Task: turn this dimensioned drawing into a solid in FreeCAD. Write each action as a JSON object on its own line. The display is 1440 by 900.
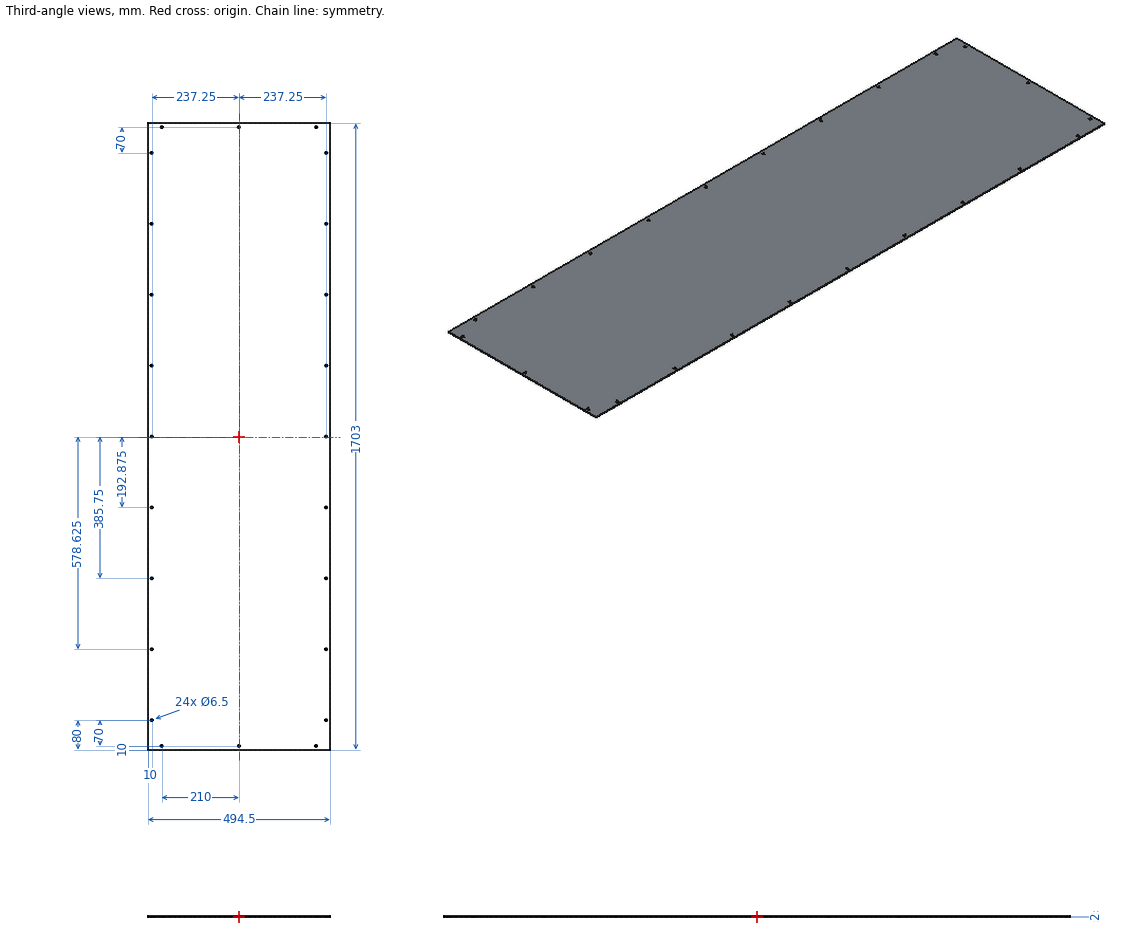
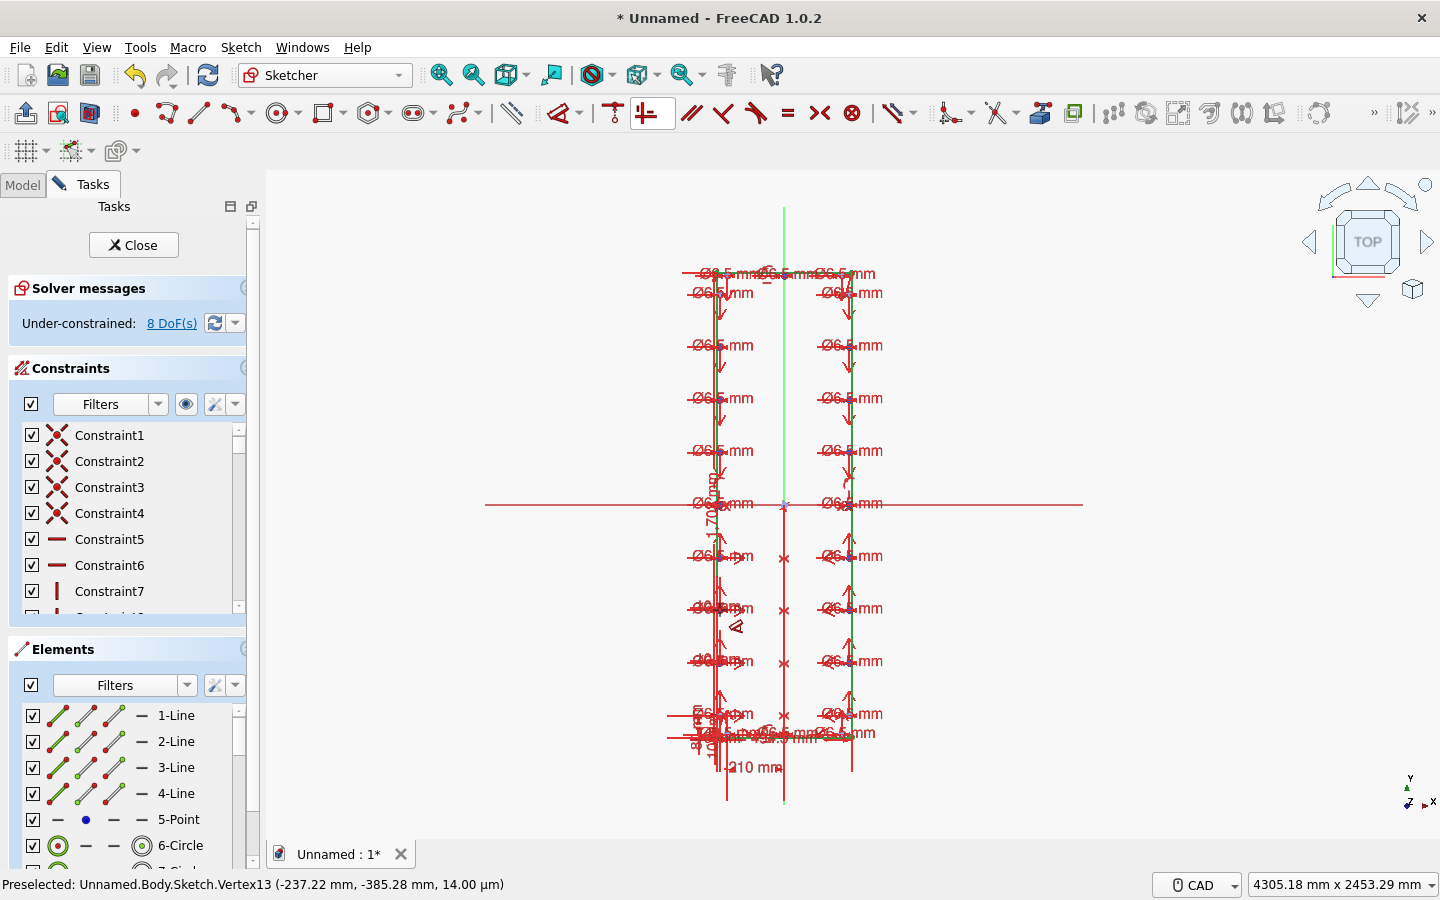
{"action": "scroll", "coordinate": [717, 738], "scroll_direction": "up", "scroll_amount": 14}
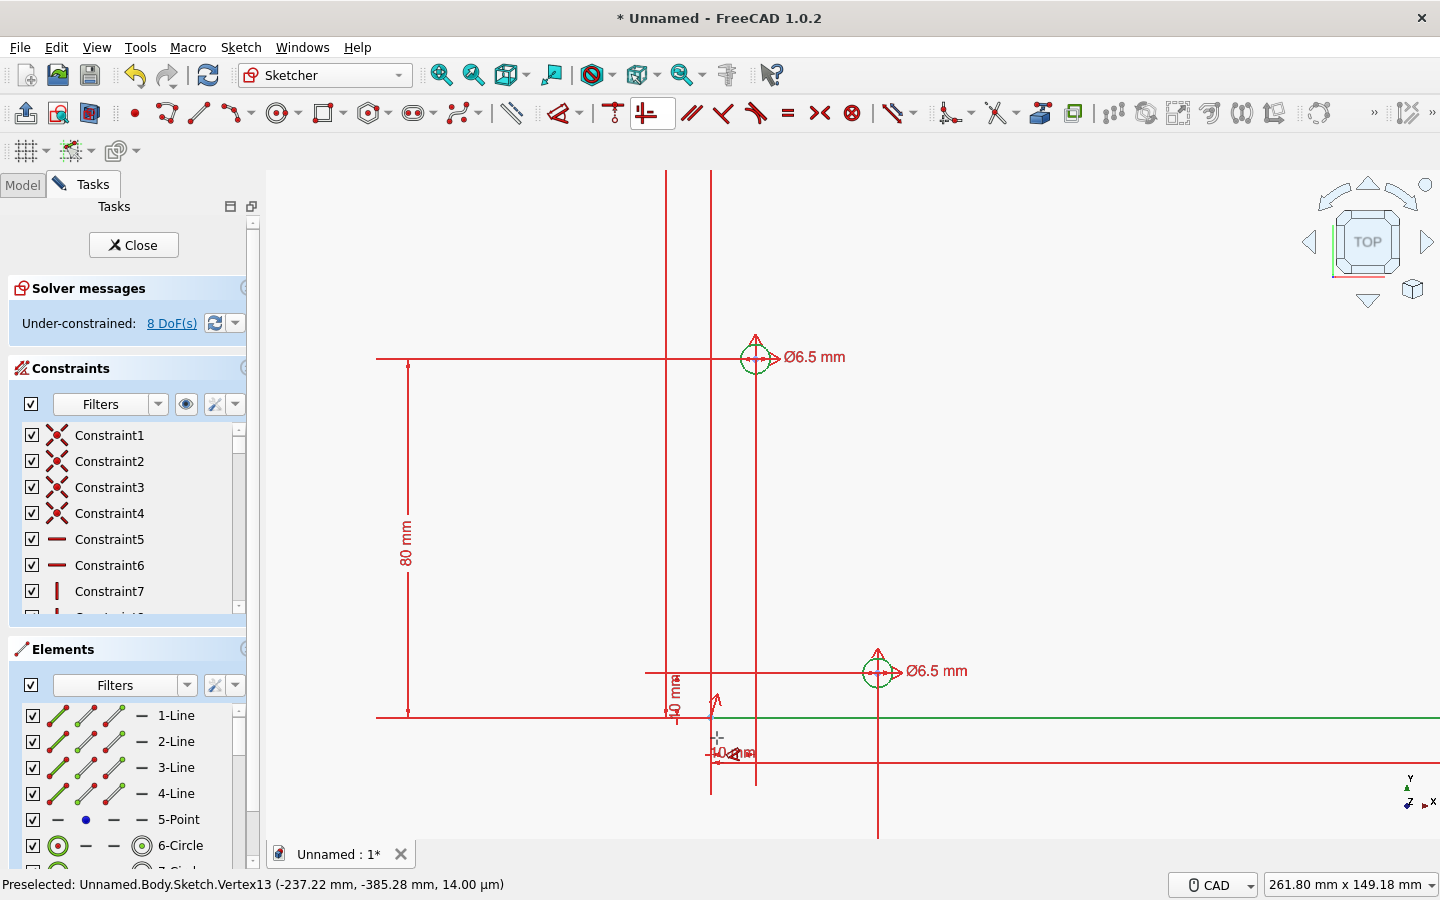
{"action": "left_click", "coordinate": [711, 718]}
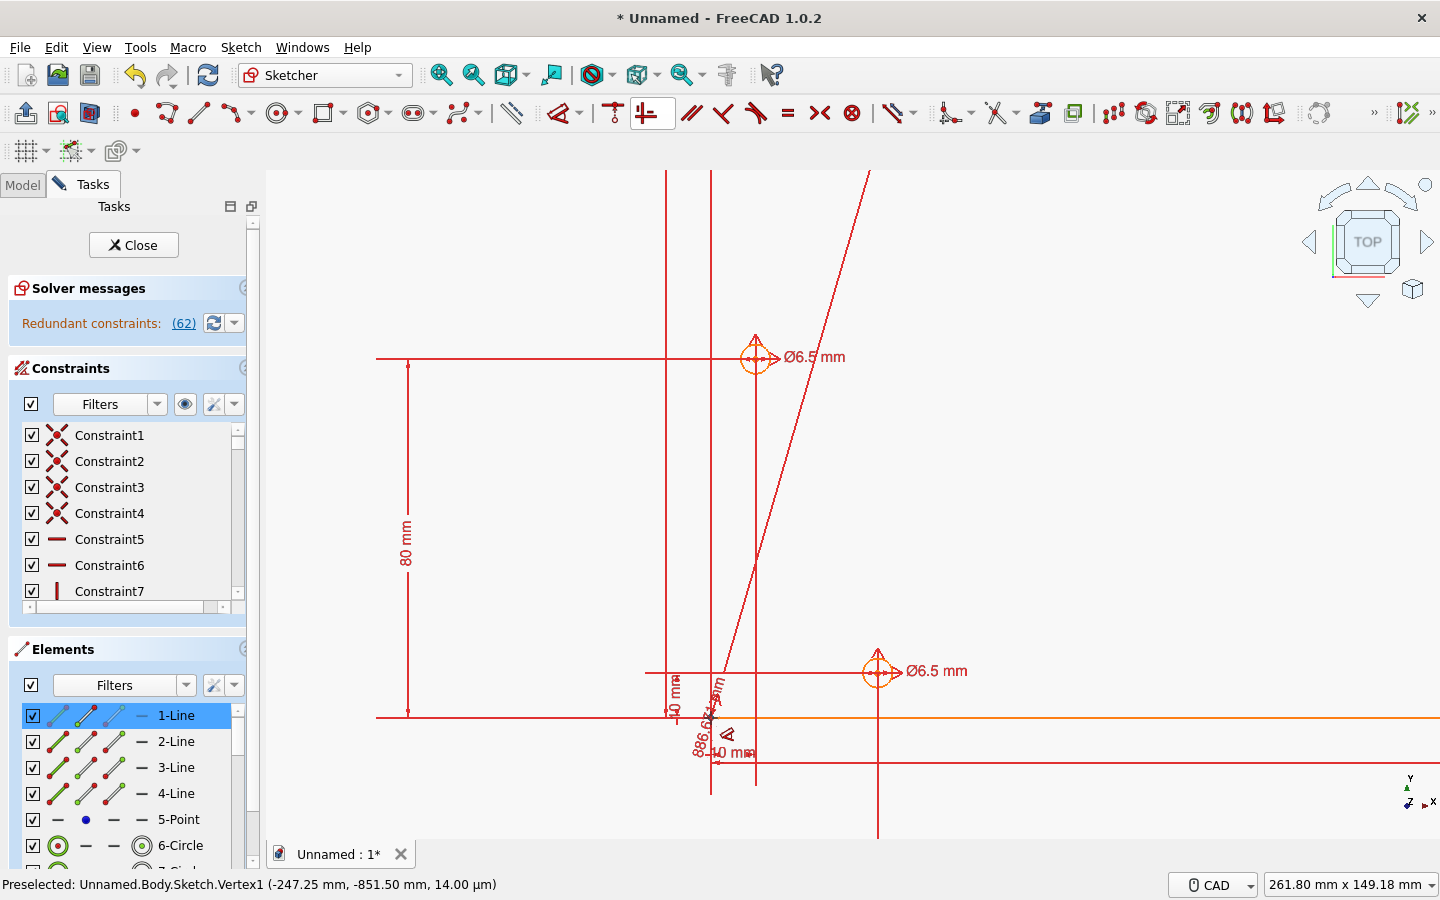
{"action": "scroll", "coordinate": [717, 738], "scroll_direction": "down", "scroll_amount": 14}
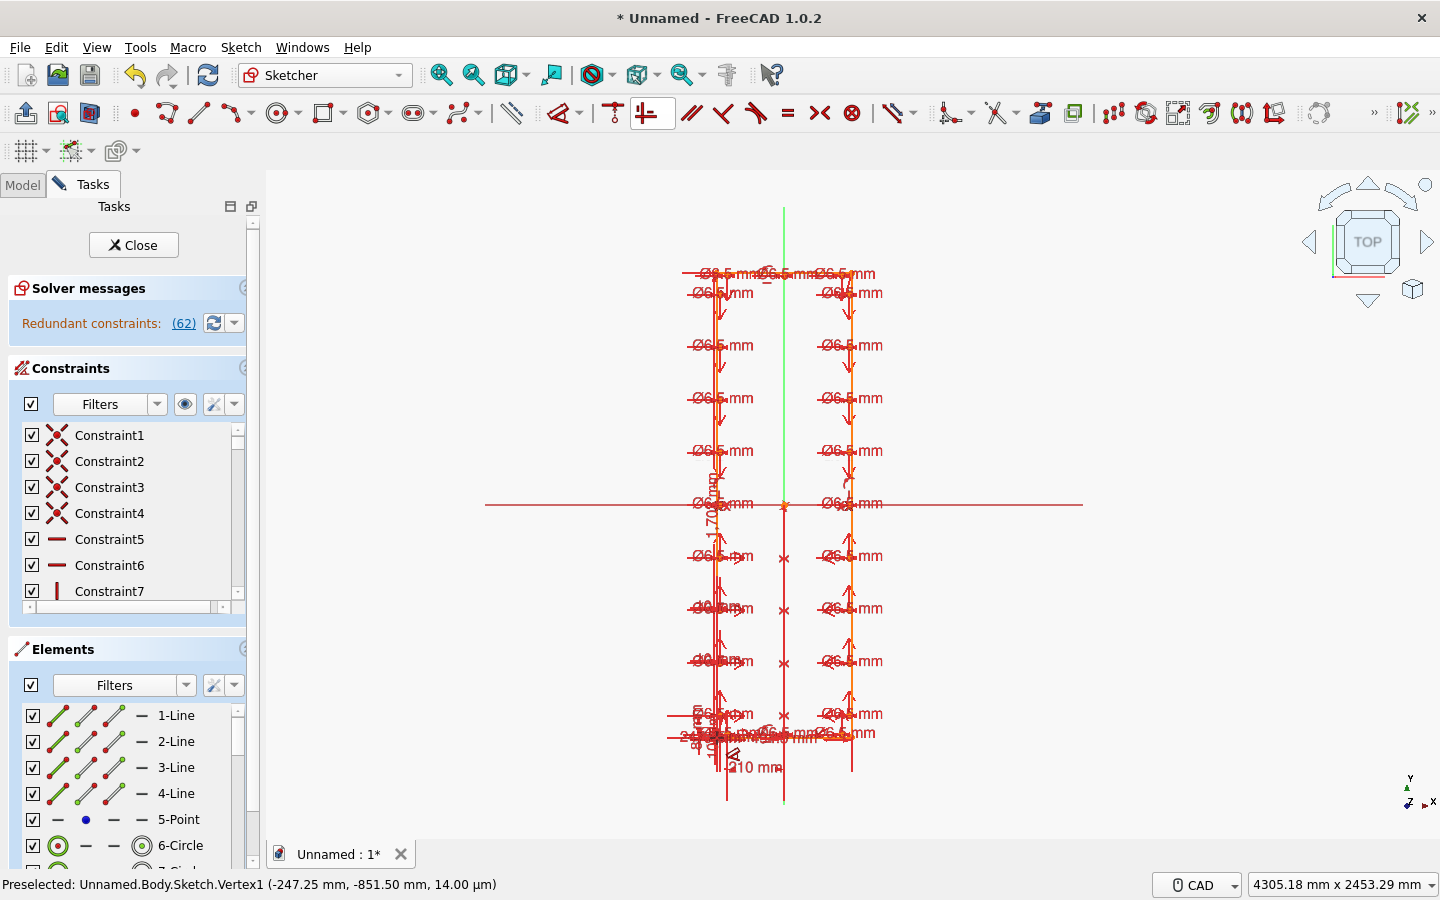
{"action": "scroll", "coordinate": [720, 558], "scroll_direction": "up", "scroll_amount": 14}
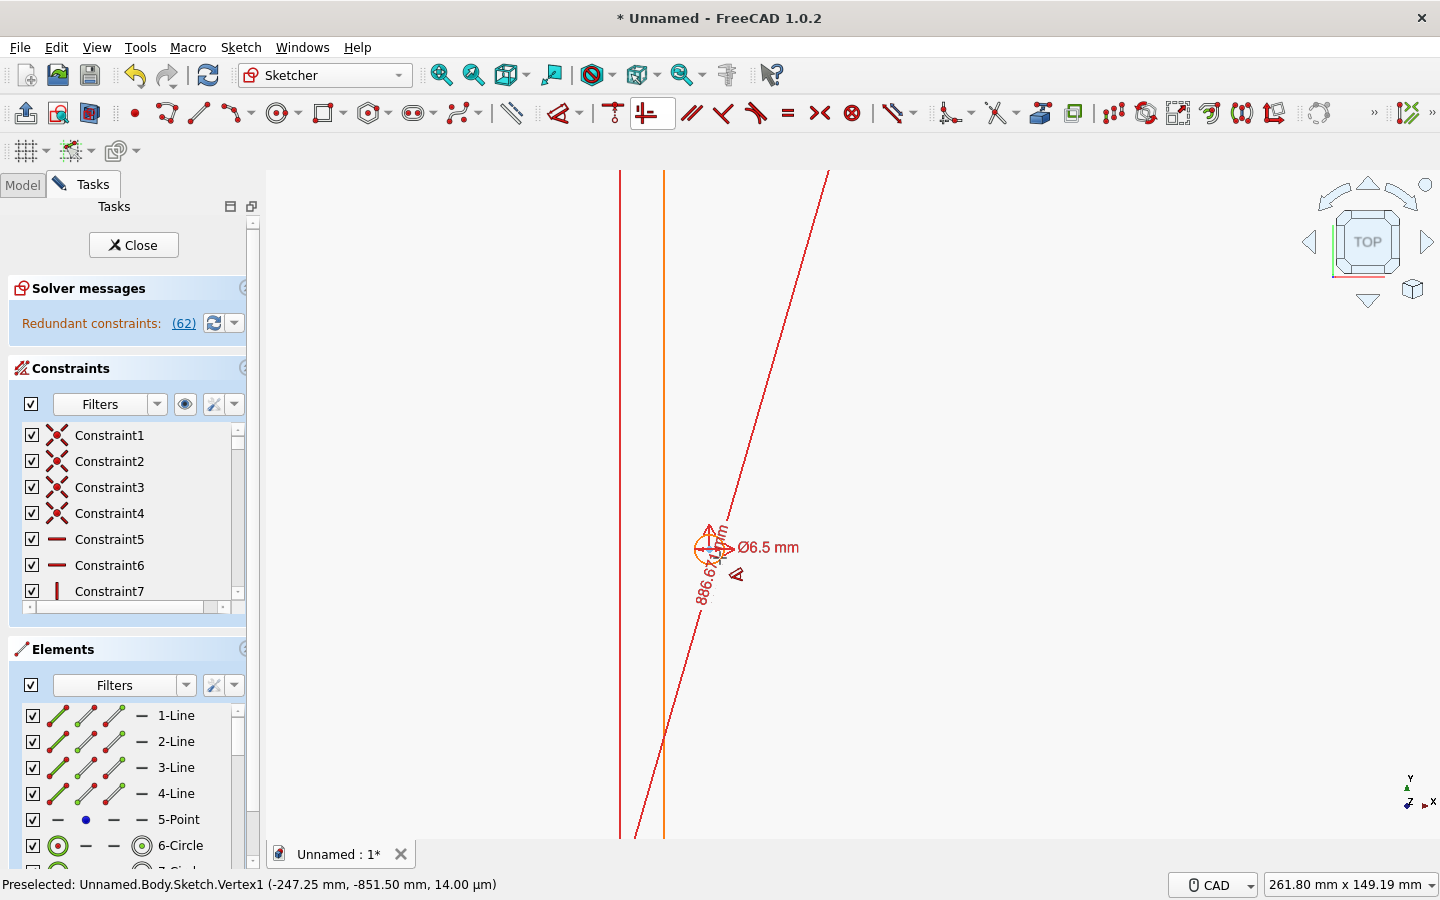
{"action": "left_click", "coordinate": [709, 549]}
{"action": "left_click", "coordinate": [687, 515]}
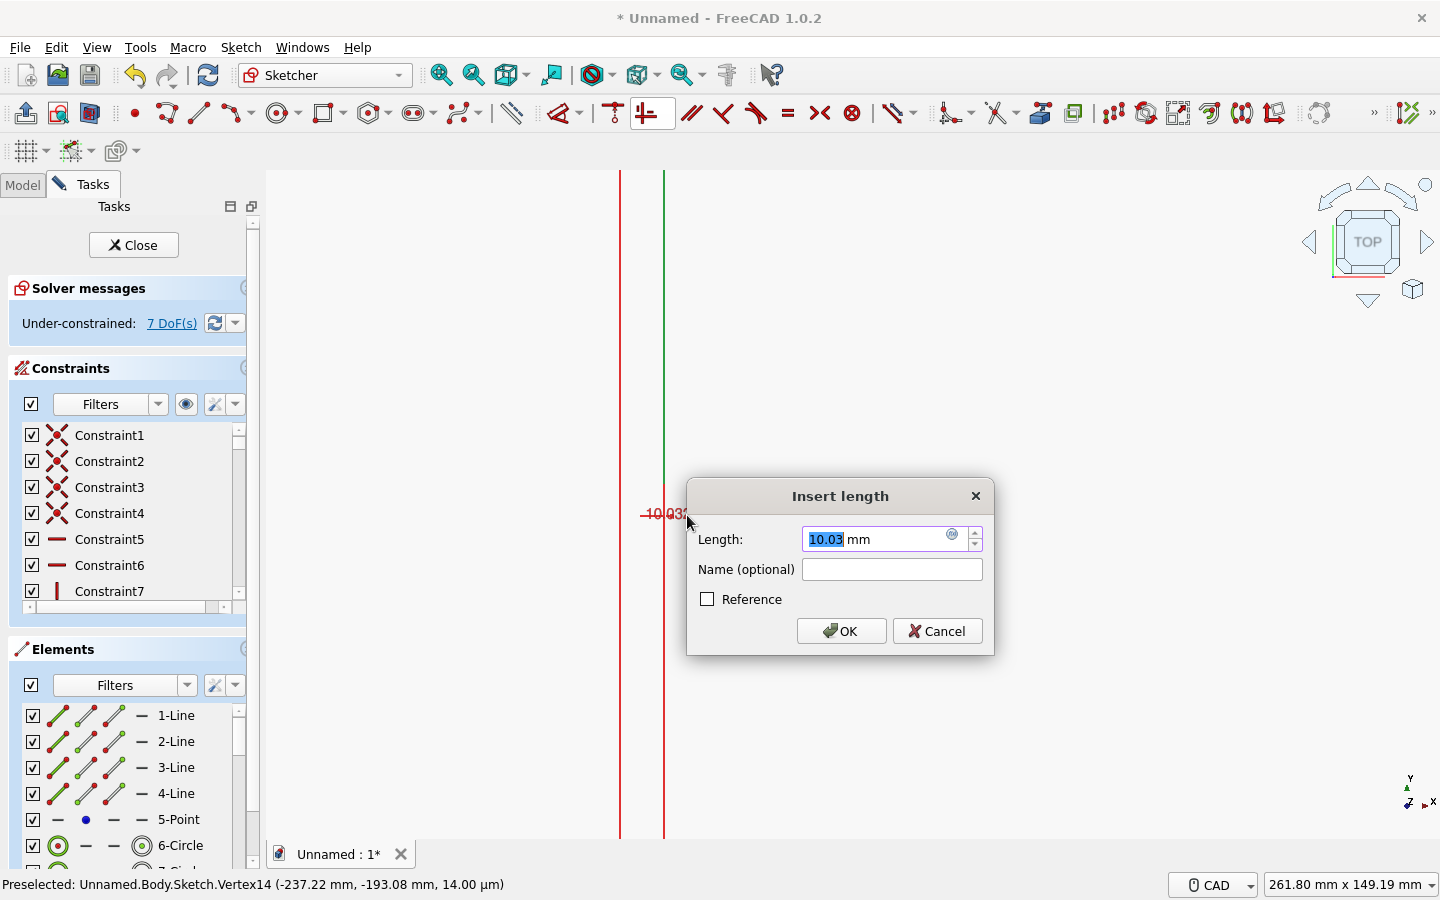
{"action": "type", "text": "10"}
{"action": "key", "text": "Return"}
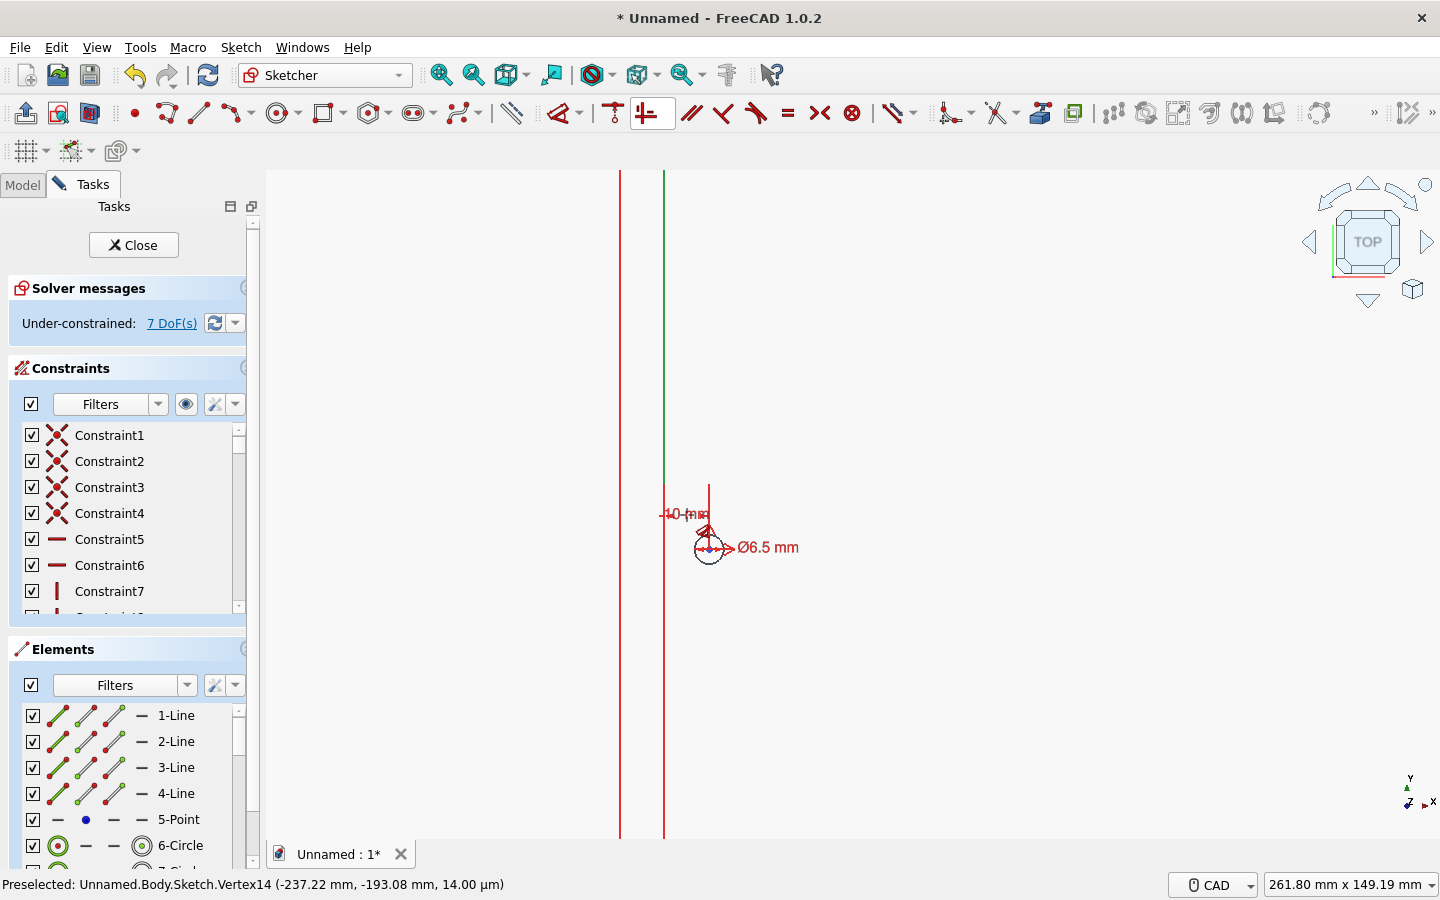
{"action": "scroll", "coordinate": [720, 558], "scroll_direction": "down", "scroll_amount": 14}